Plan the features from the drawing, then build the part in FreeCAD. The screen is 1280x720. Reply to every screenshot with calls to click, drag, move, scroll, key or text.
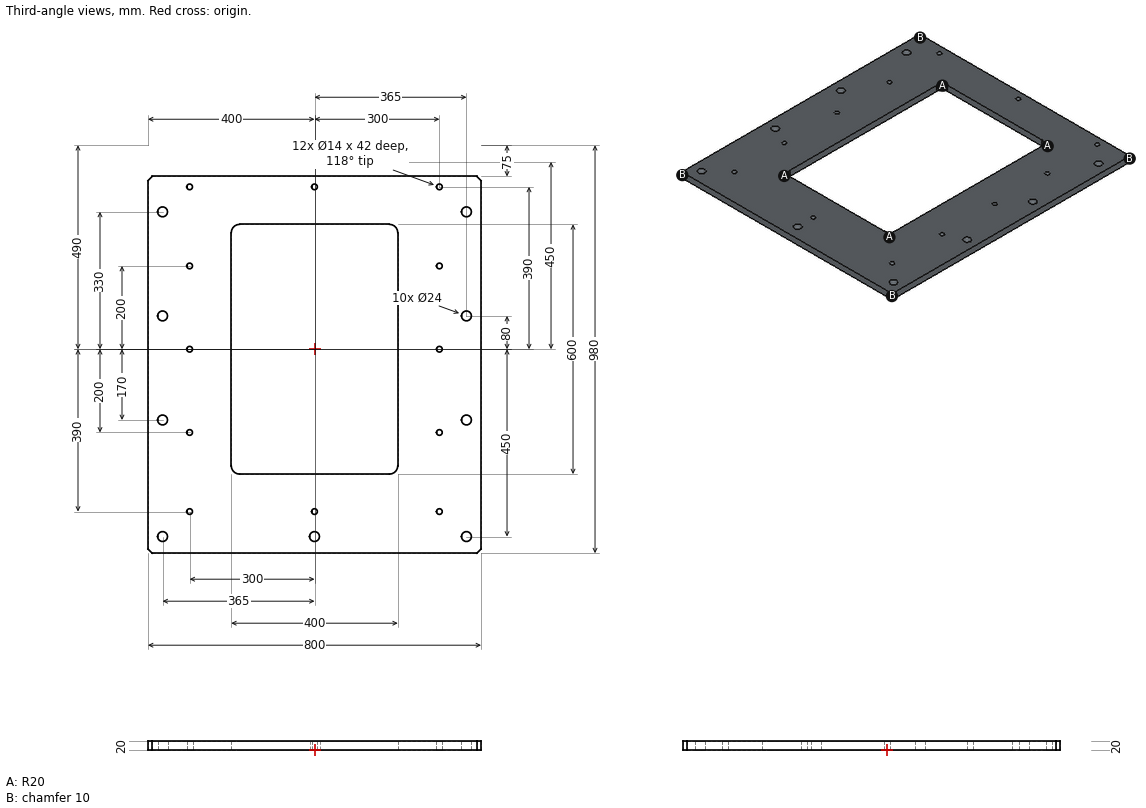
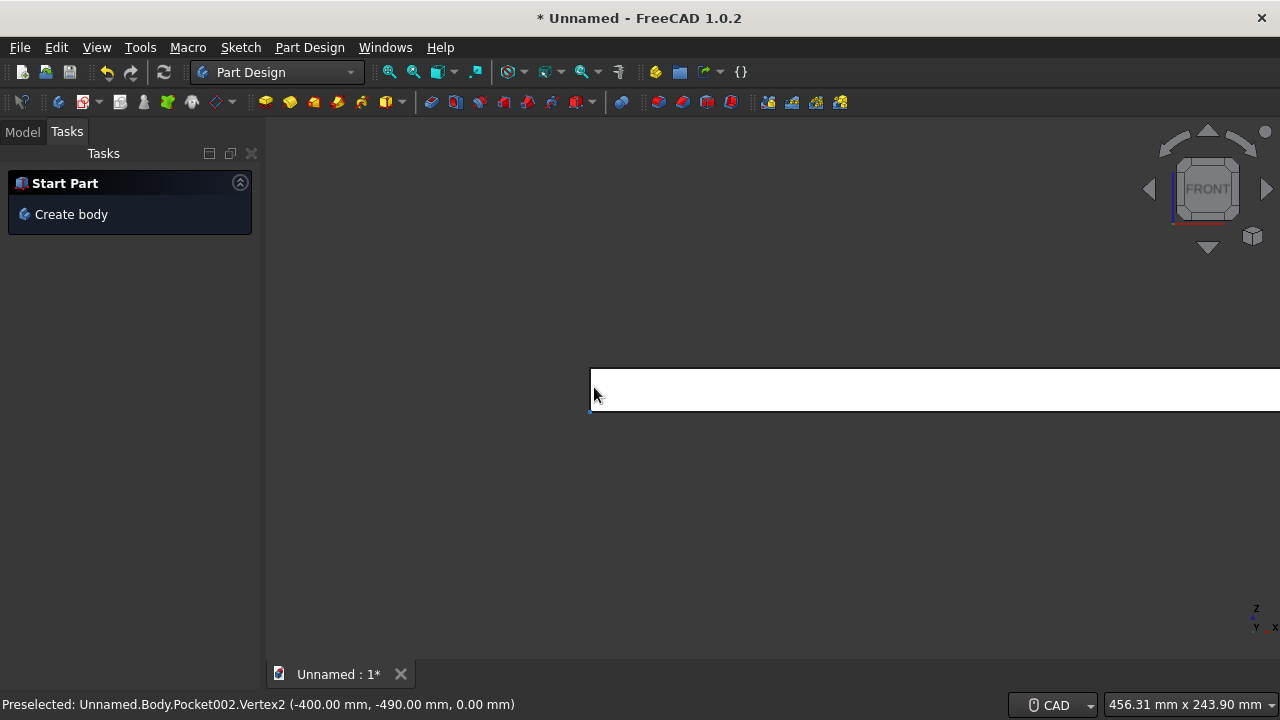
click(590, 389)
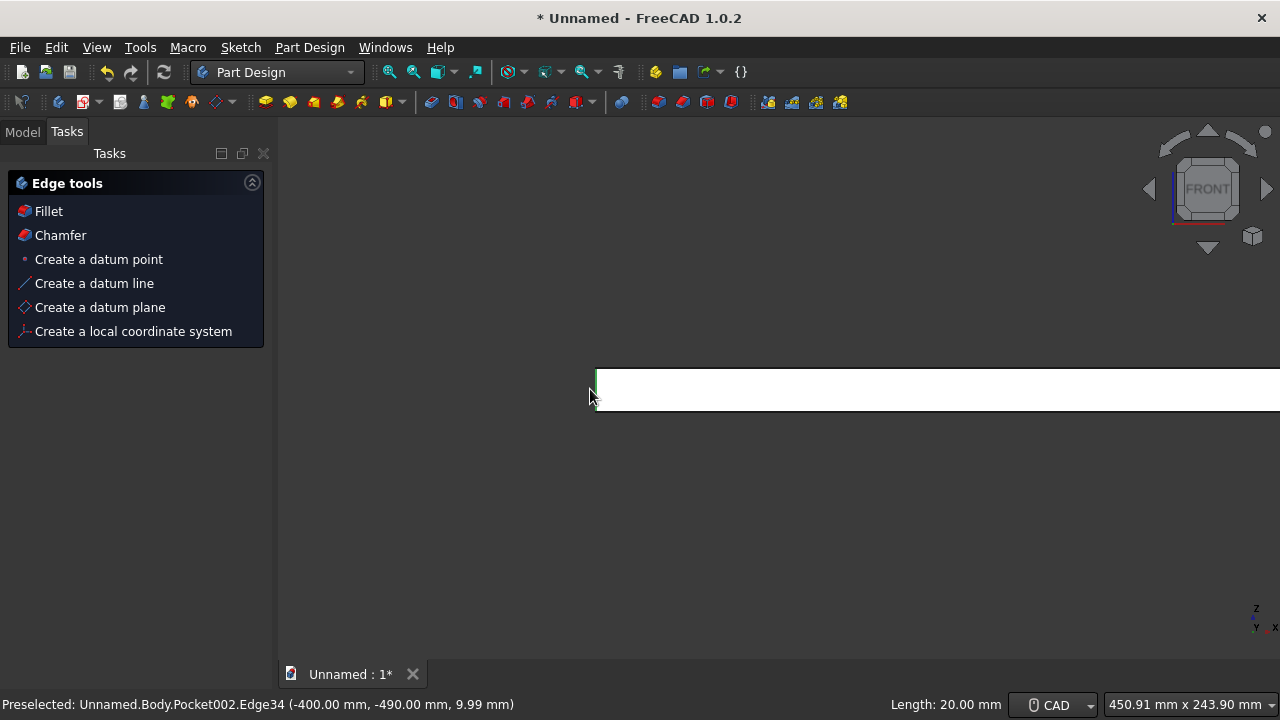
click(390, 72)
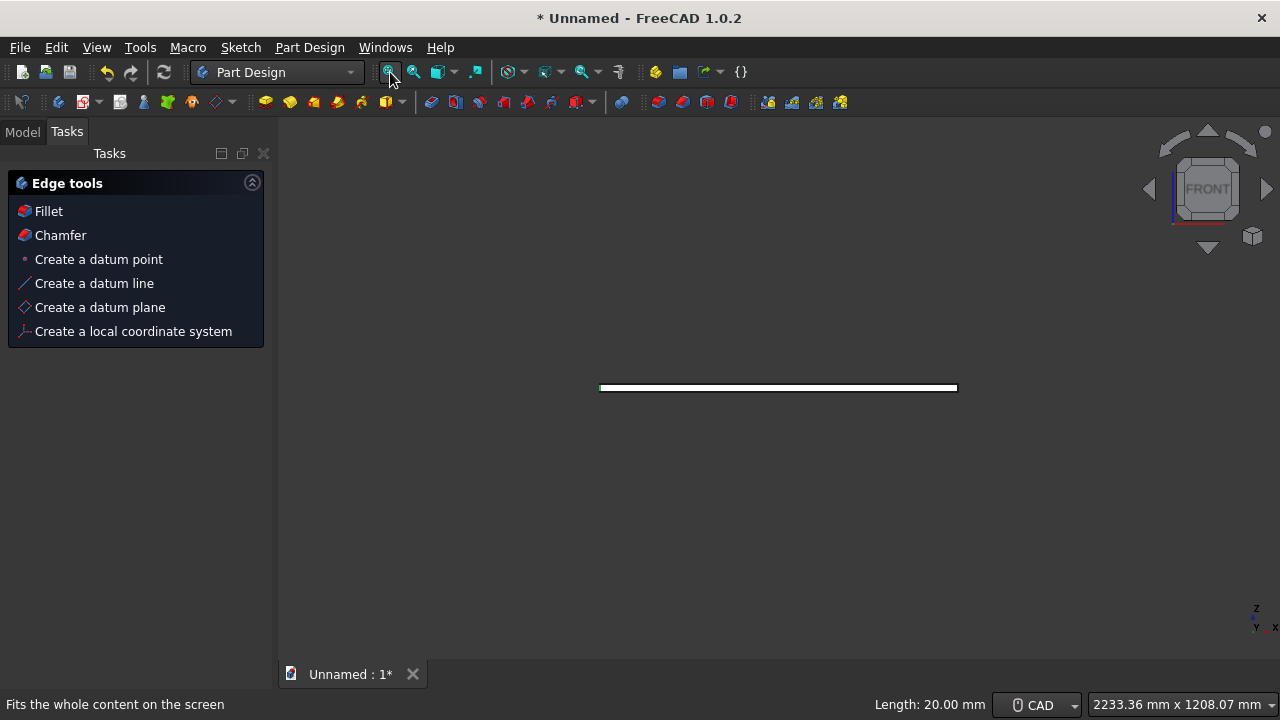
key(3)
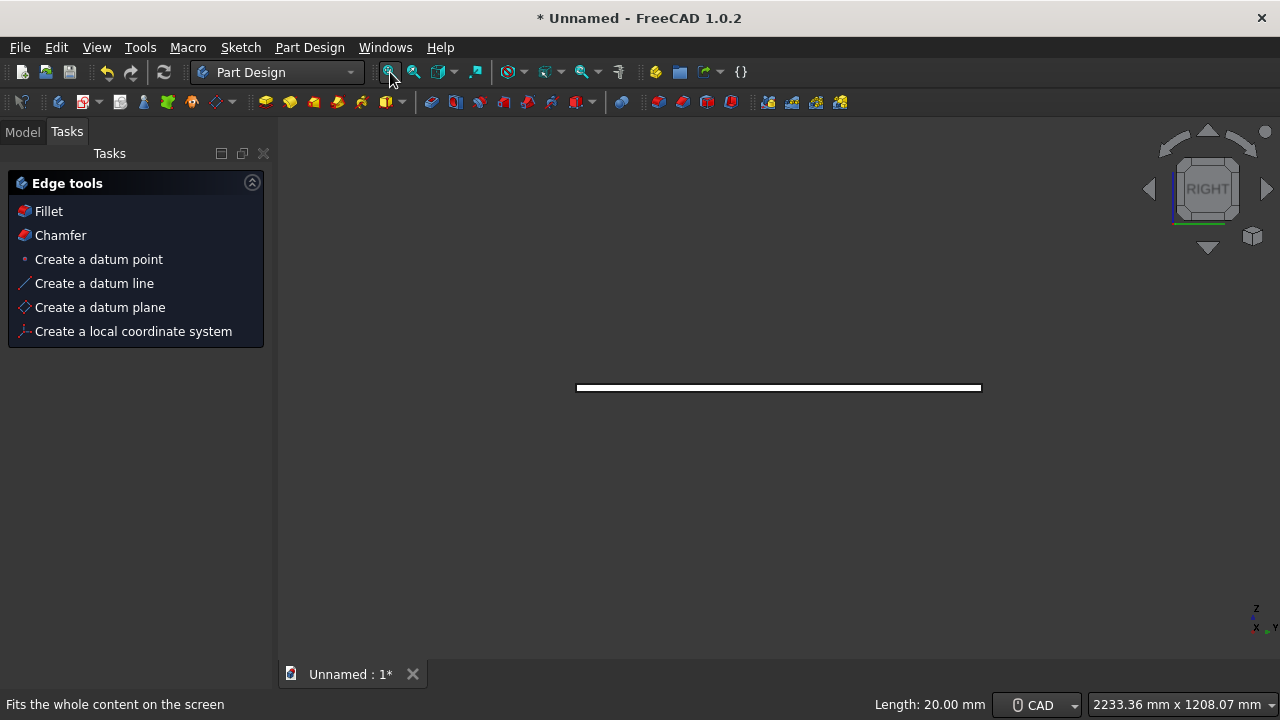
click(390, 72)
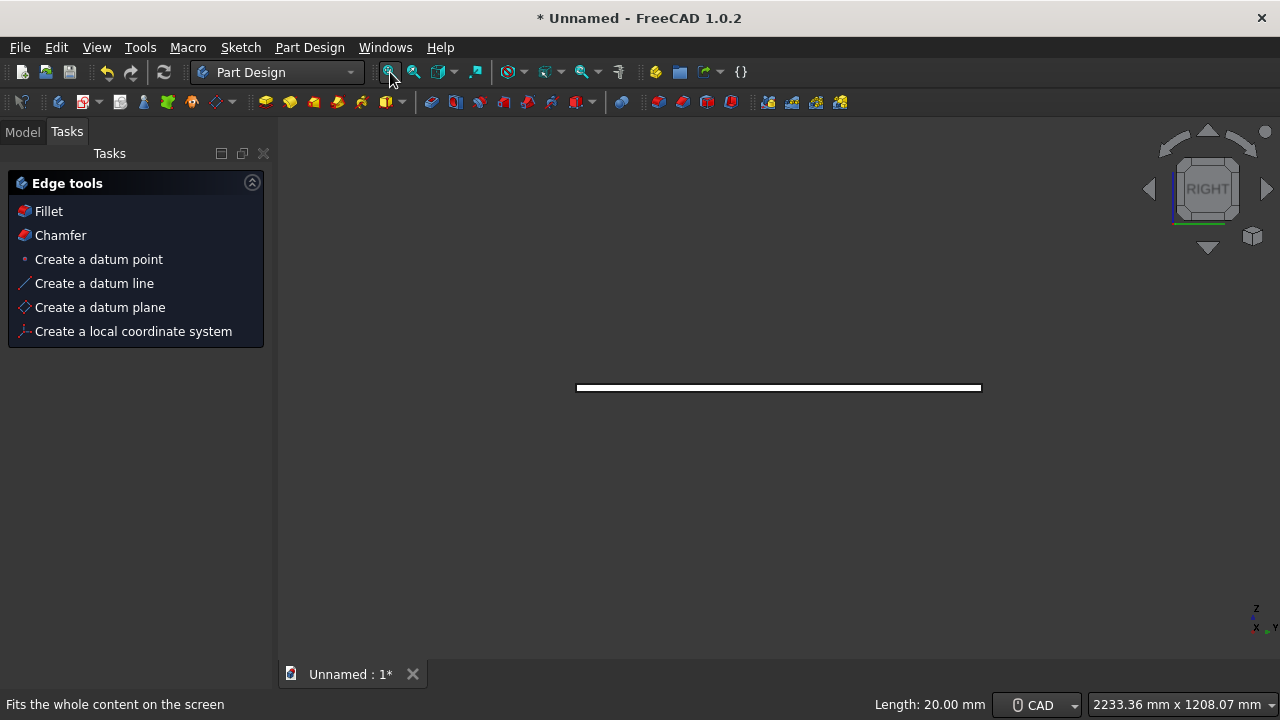
scroll(982, 387, up, 8)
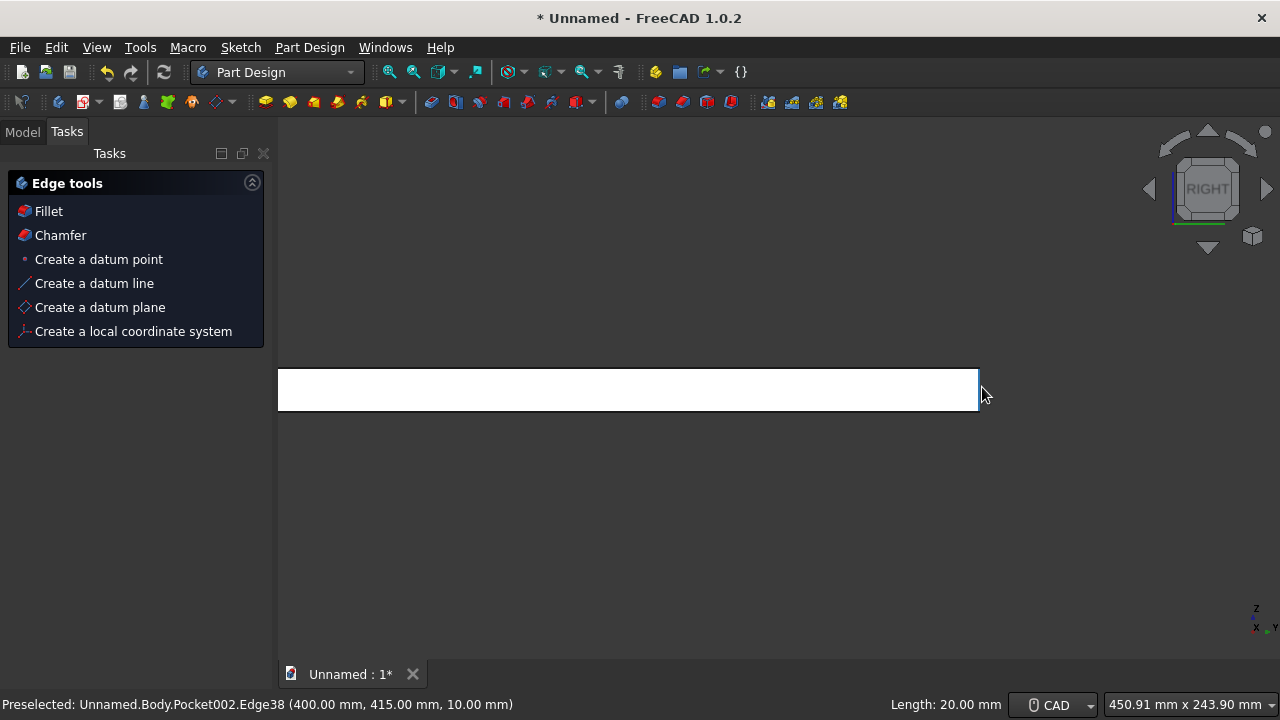
click(979, 389, ctrl)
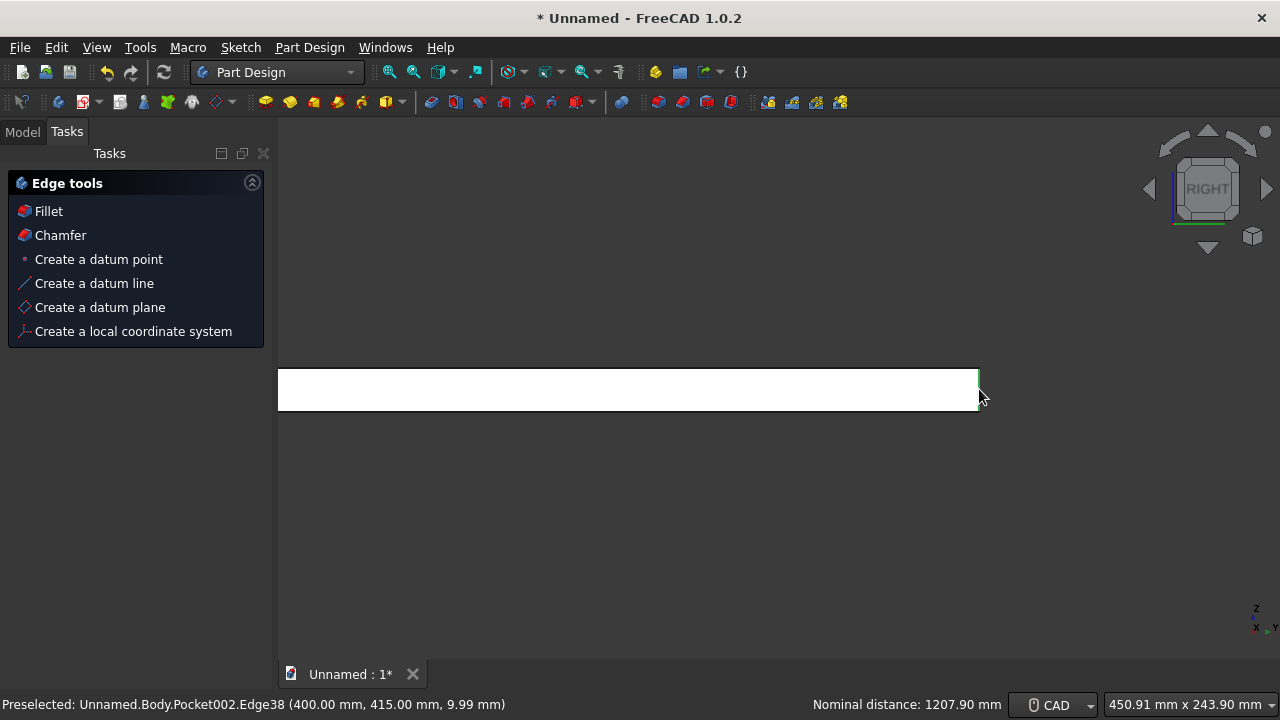
click(390, 72)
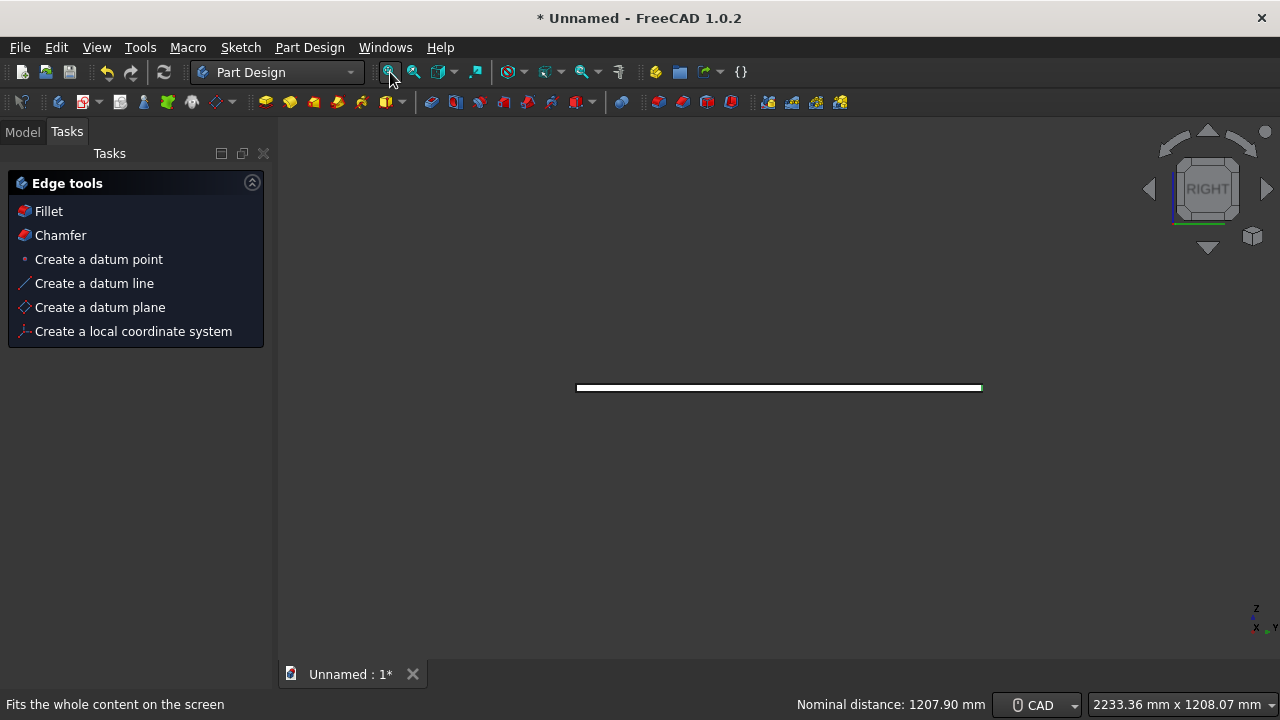
key(5)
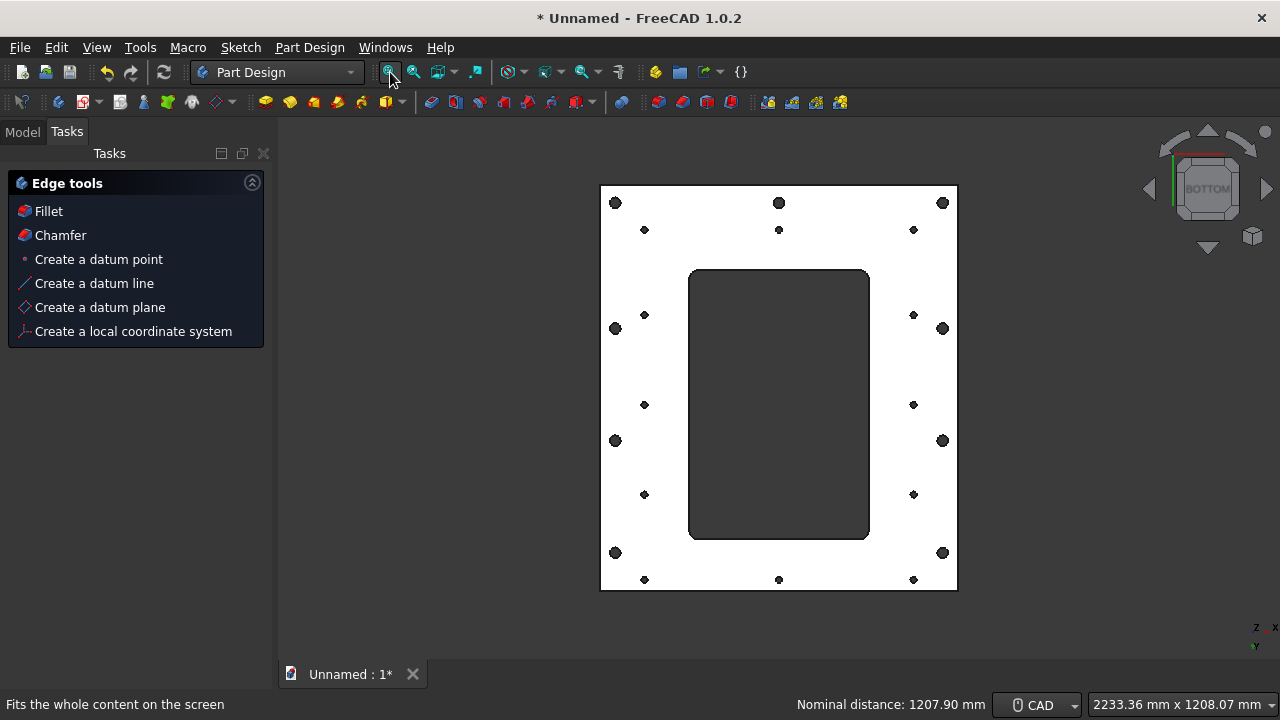
scroll(600, 590, up, 8)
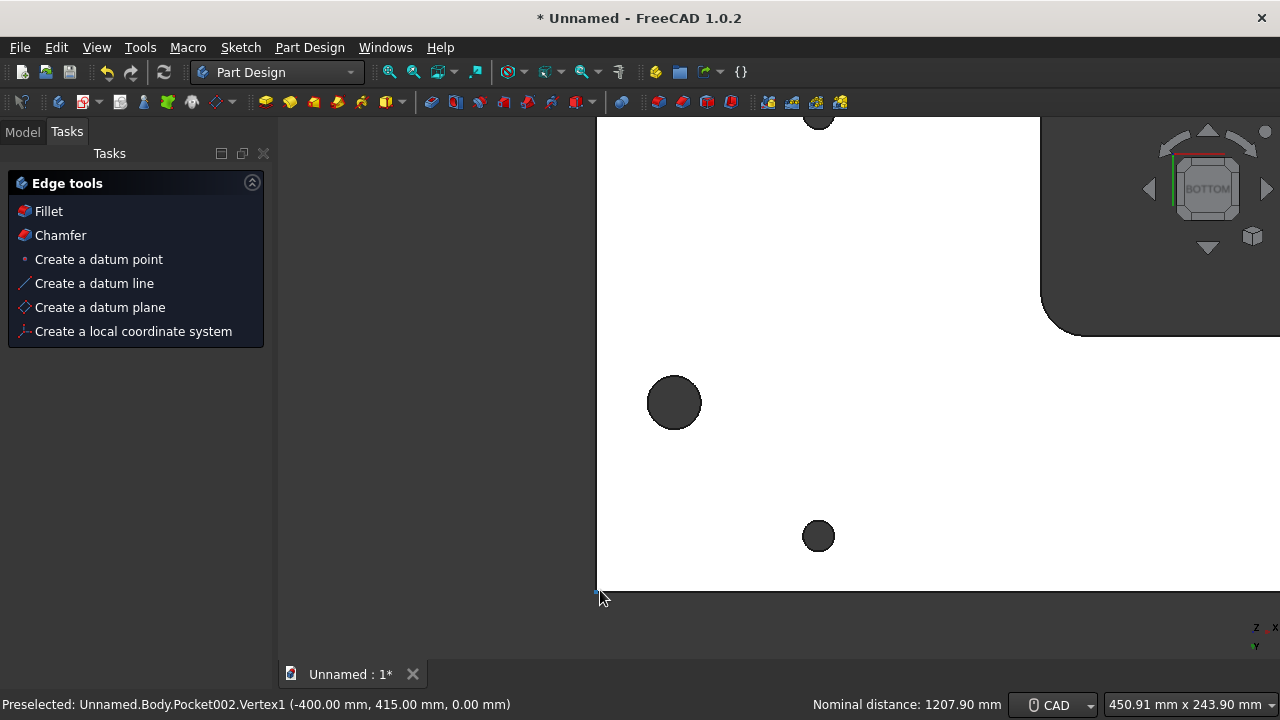
click(390, 72)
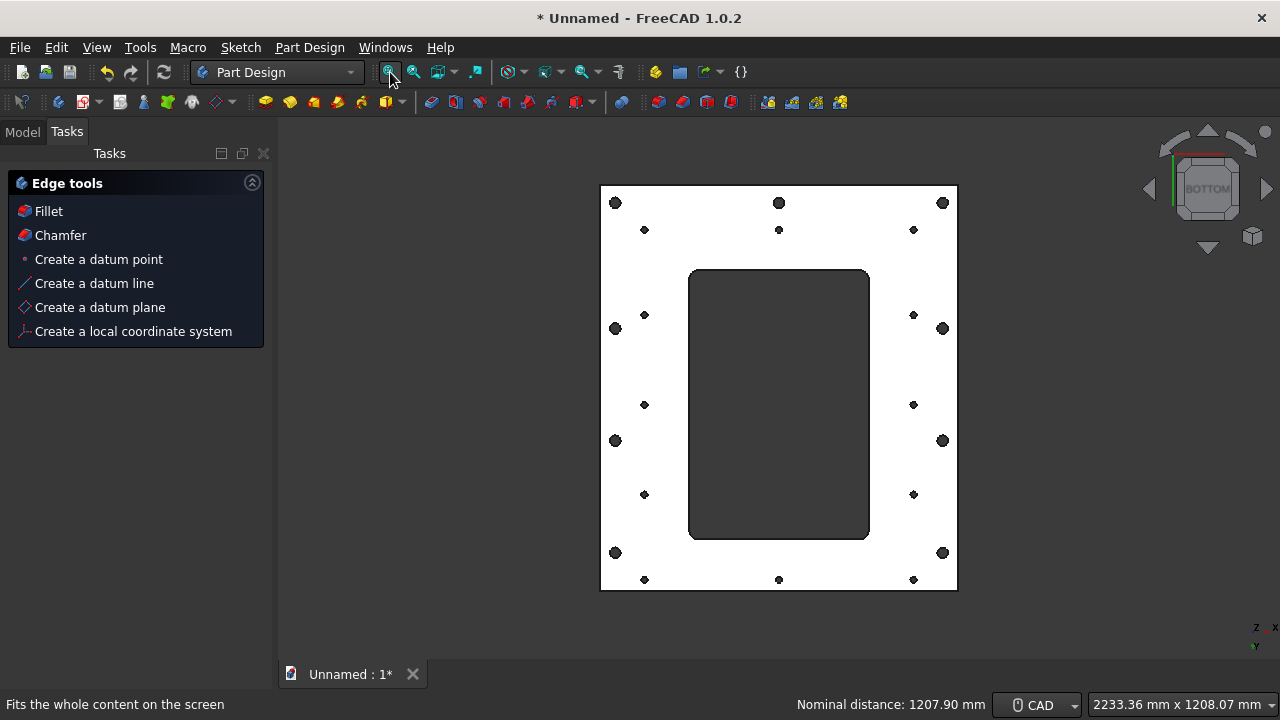
key(4)